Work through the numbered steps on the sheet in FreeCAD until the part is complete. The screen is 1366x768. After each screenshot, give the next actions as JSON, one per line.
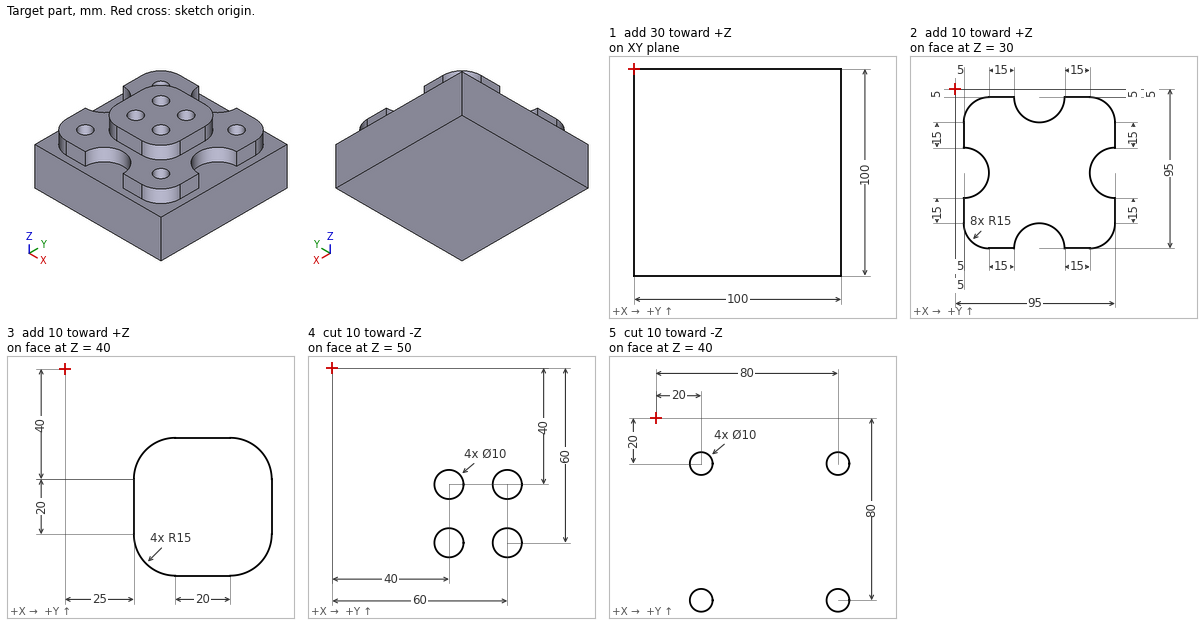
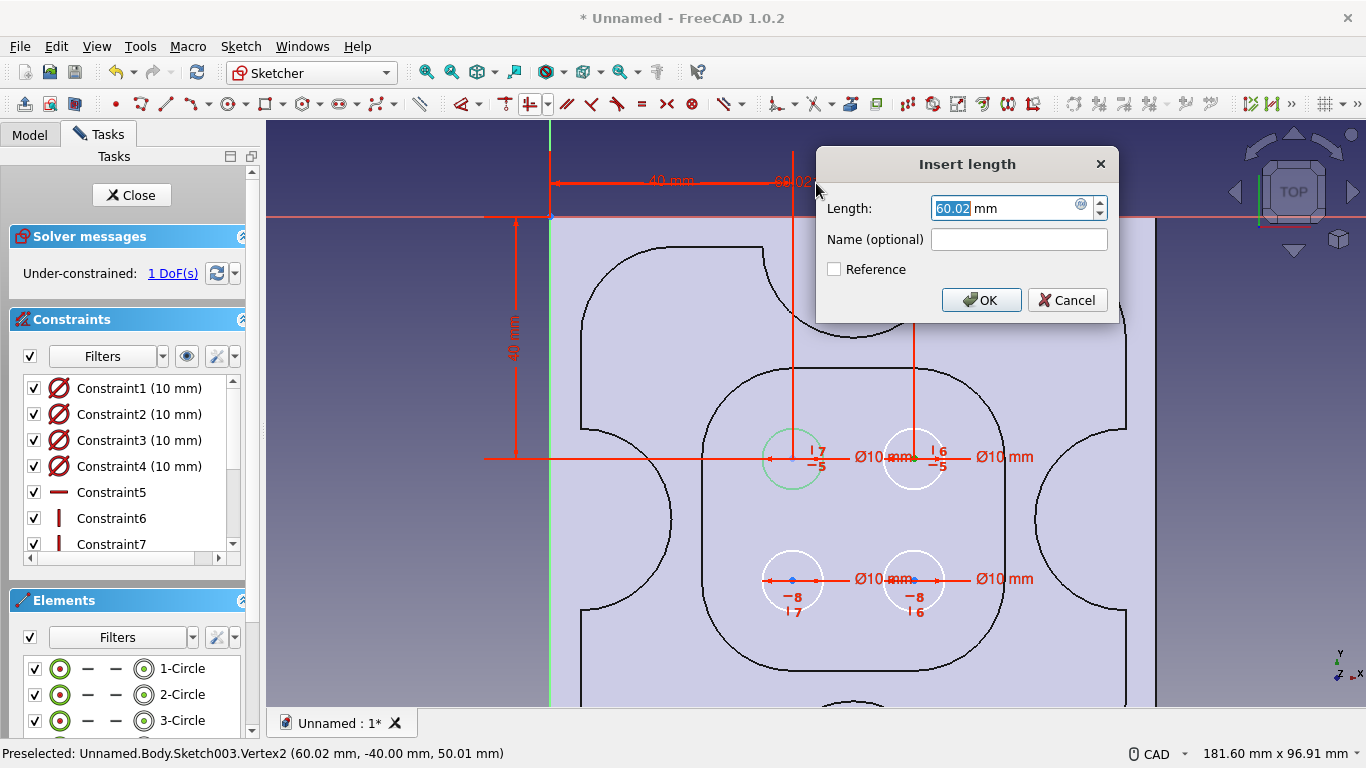
{"action": "type", "text": "60"}
{"action": "key", "text": "Return"}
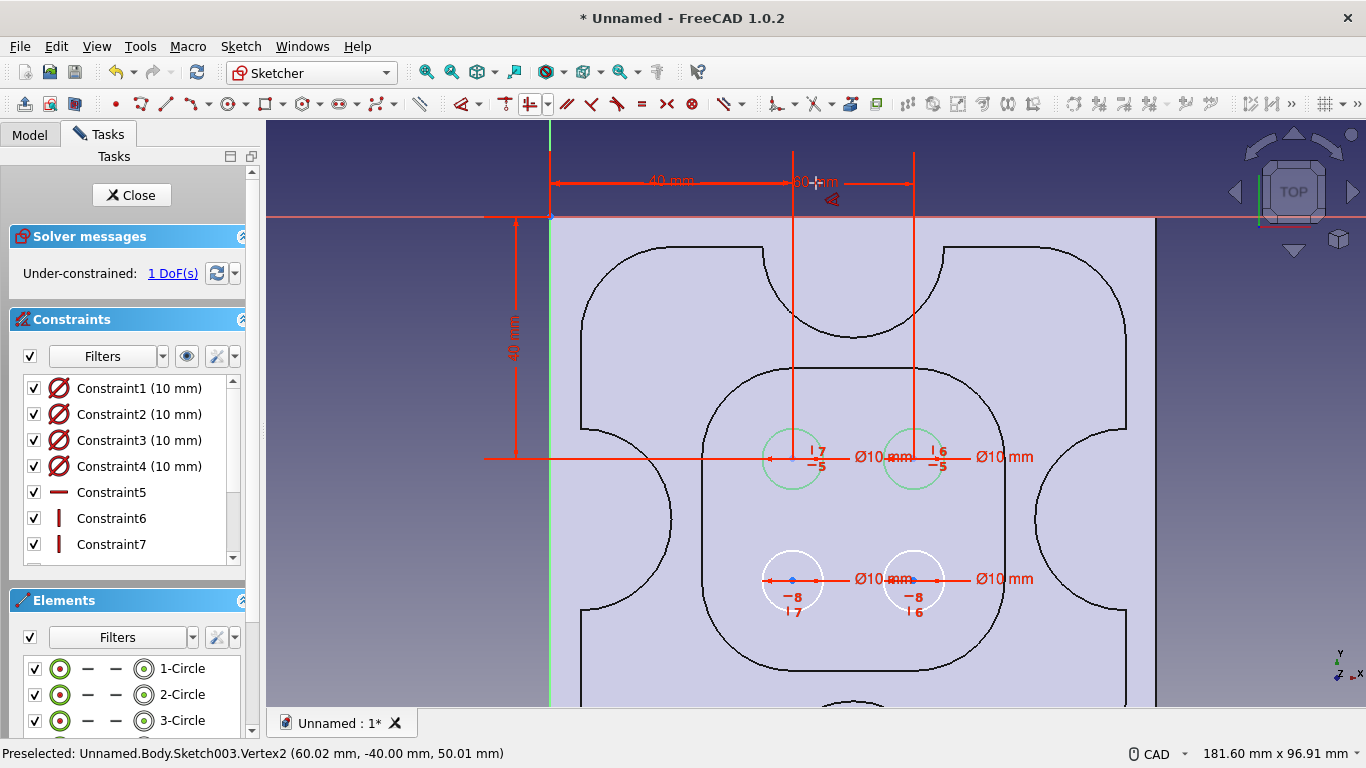
{"action": "left_click", "coordinate": [914, 581]}
{"action": "left_click", "coordinate": [516, 399]}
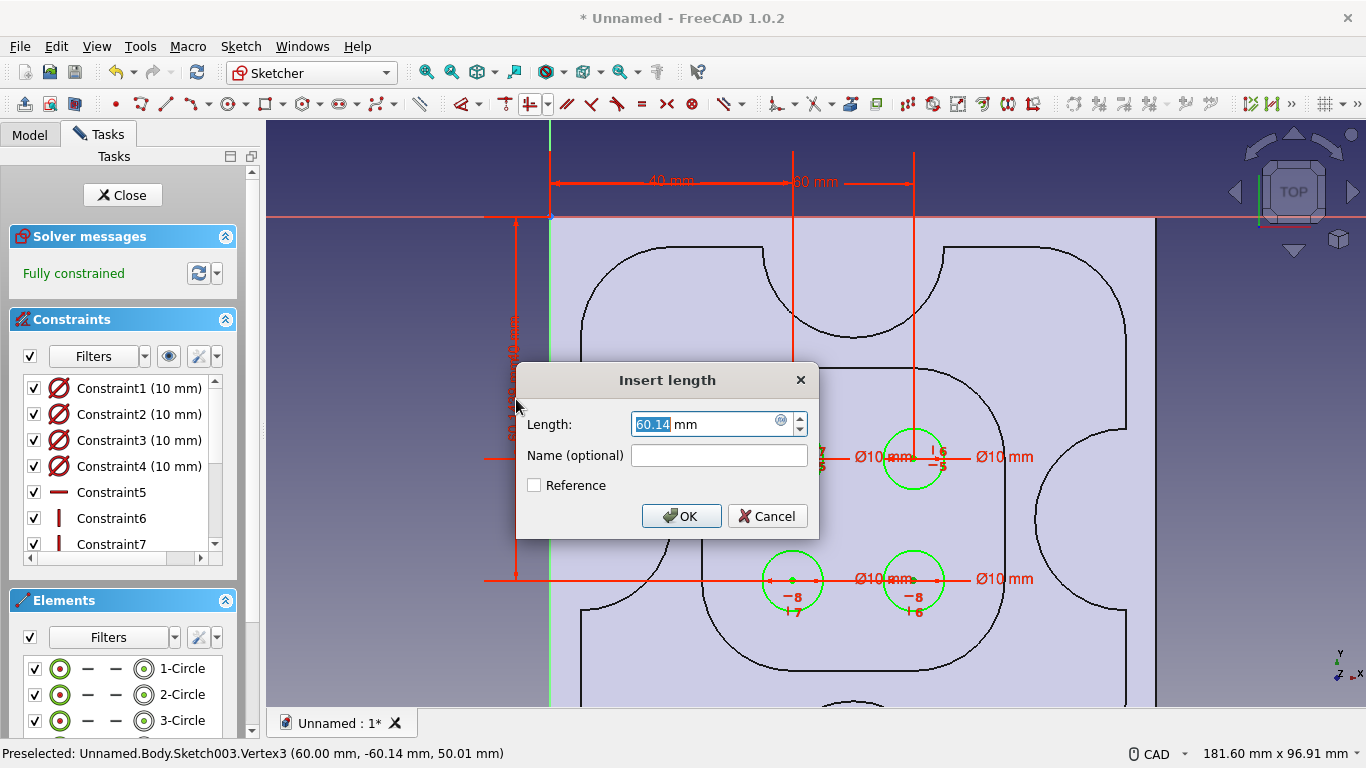
{"action": "type", "text": "60"}
{"action": "key", "text": "Return"}
{"action": "key", "text": "Escape"}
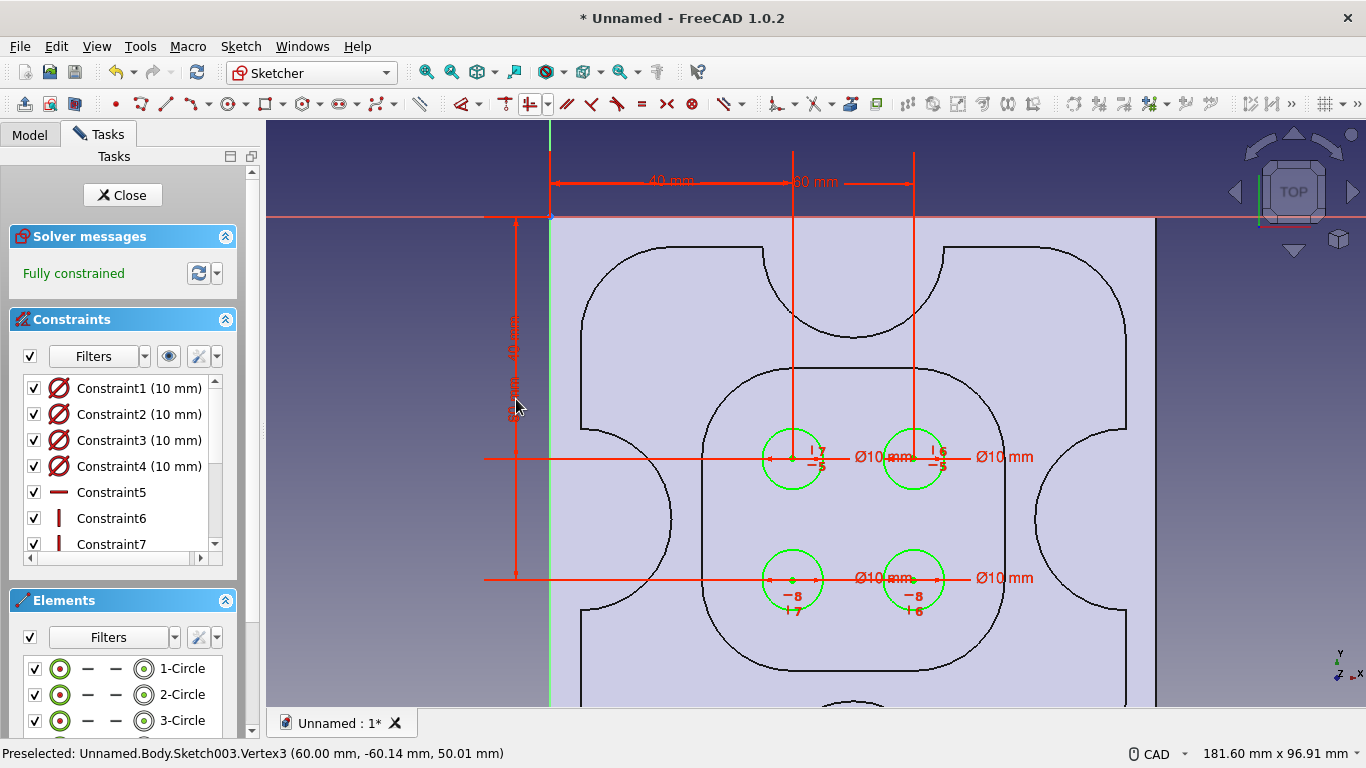
{"action": "left_click", "coordinate": [123, 195]}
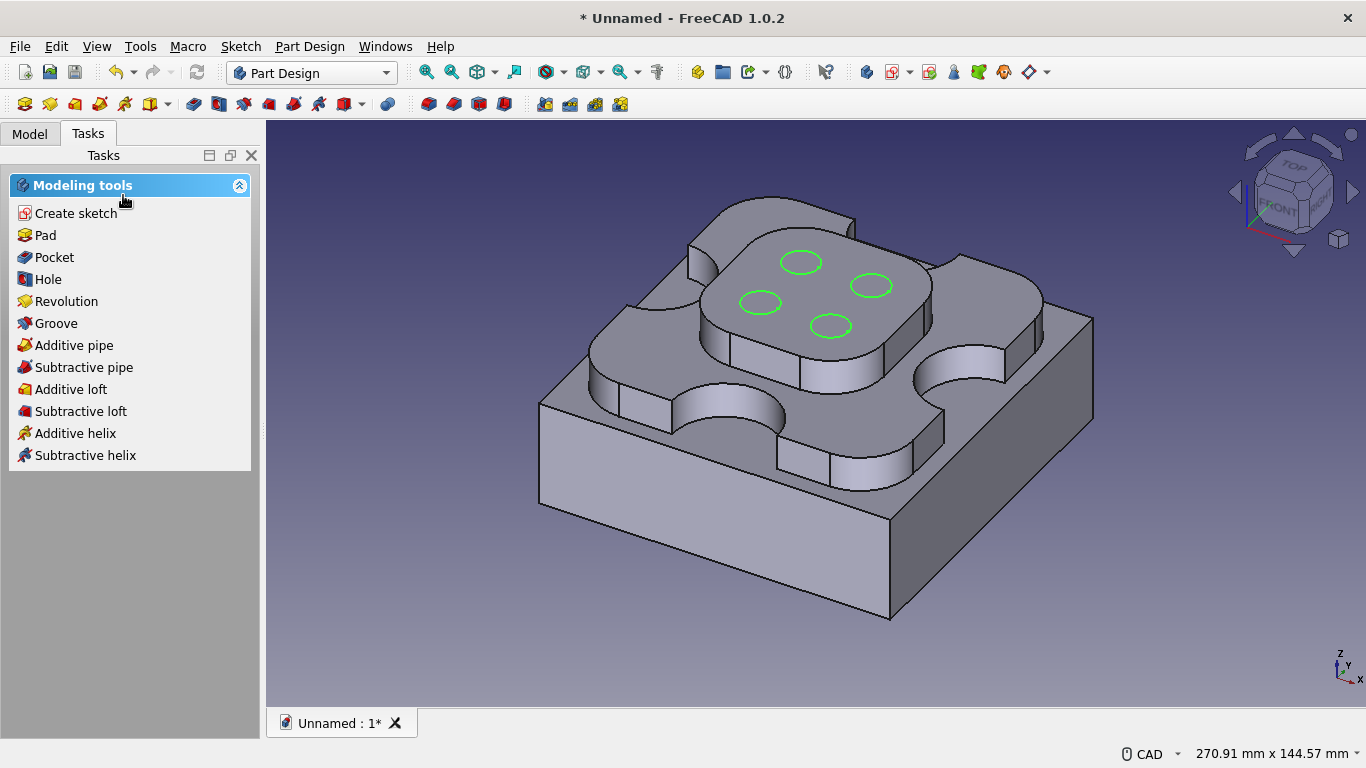
{"action": "left_click", "coordinate": [194, 104]}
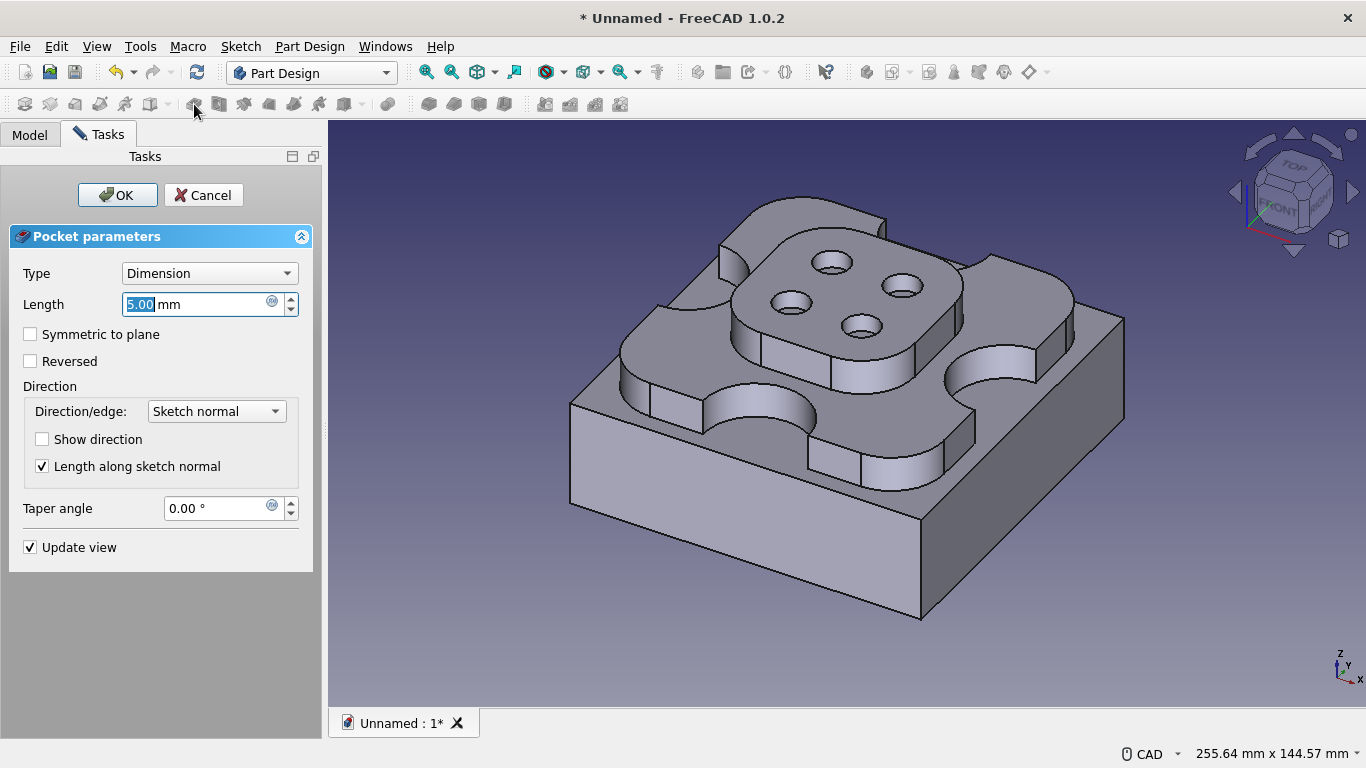
{"action": "type", "text": "10"}
{"action": "key", "text": "Tab"}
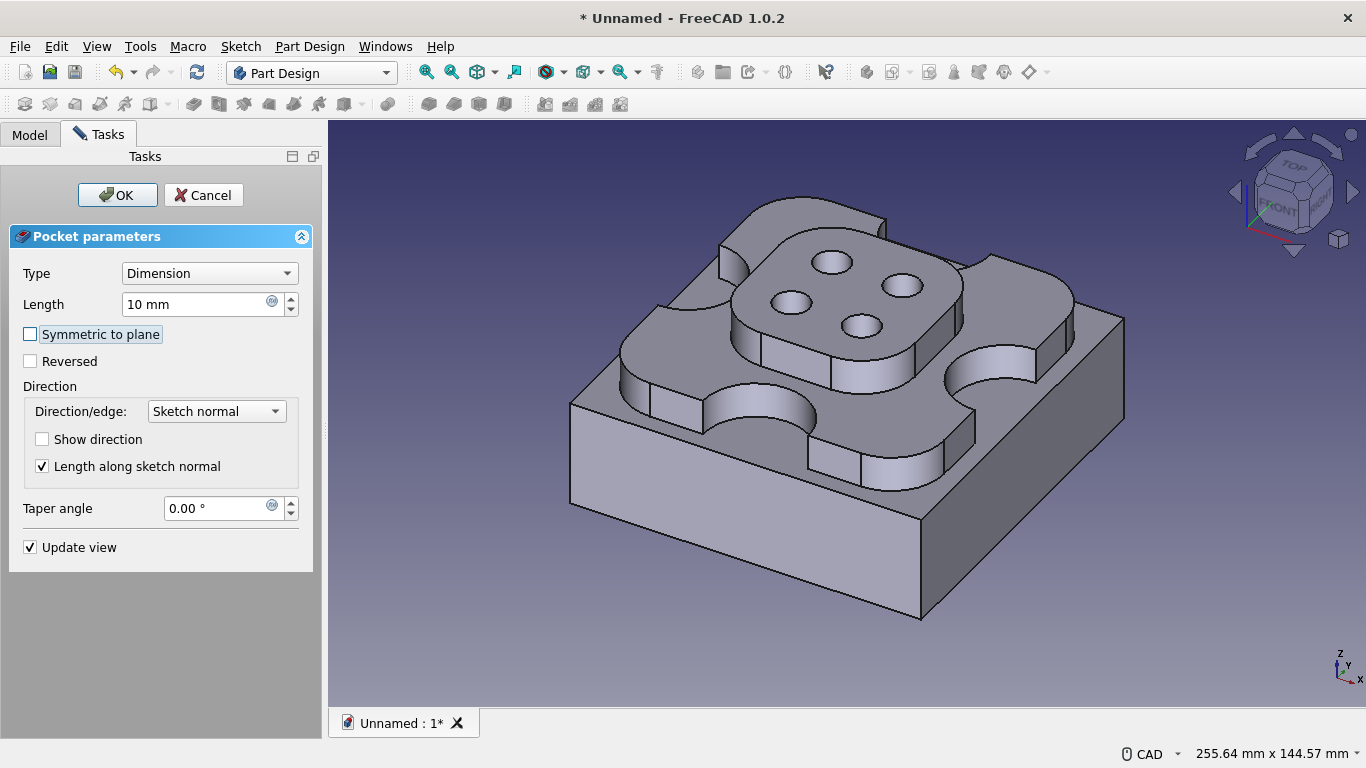
{"action": "left_click", "coordinate": [118, 195]}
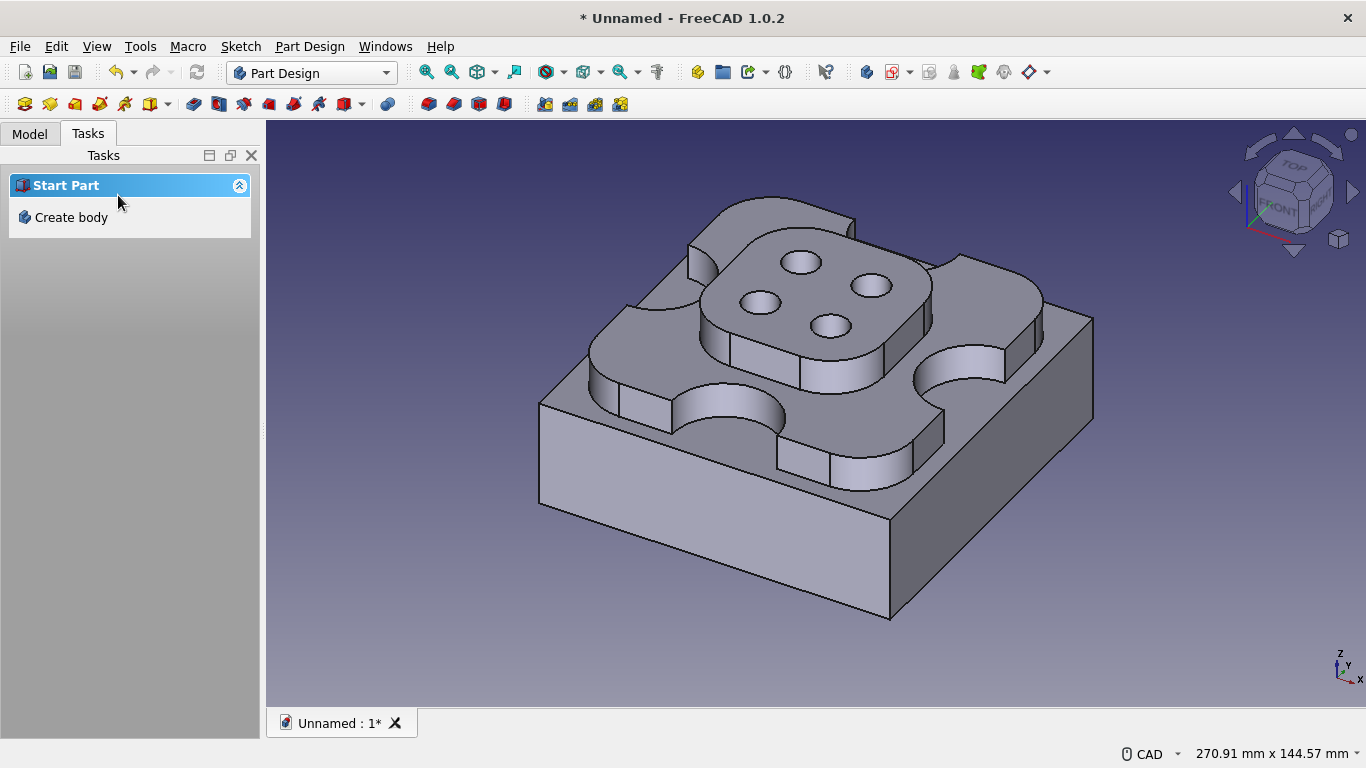
{"action": "left_click", "coordinate": [959, 305]}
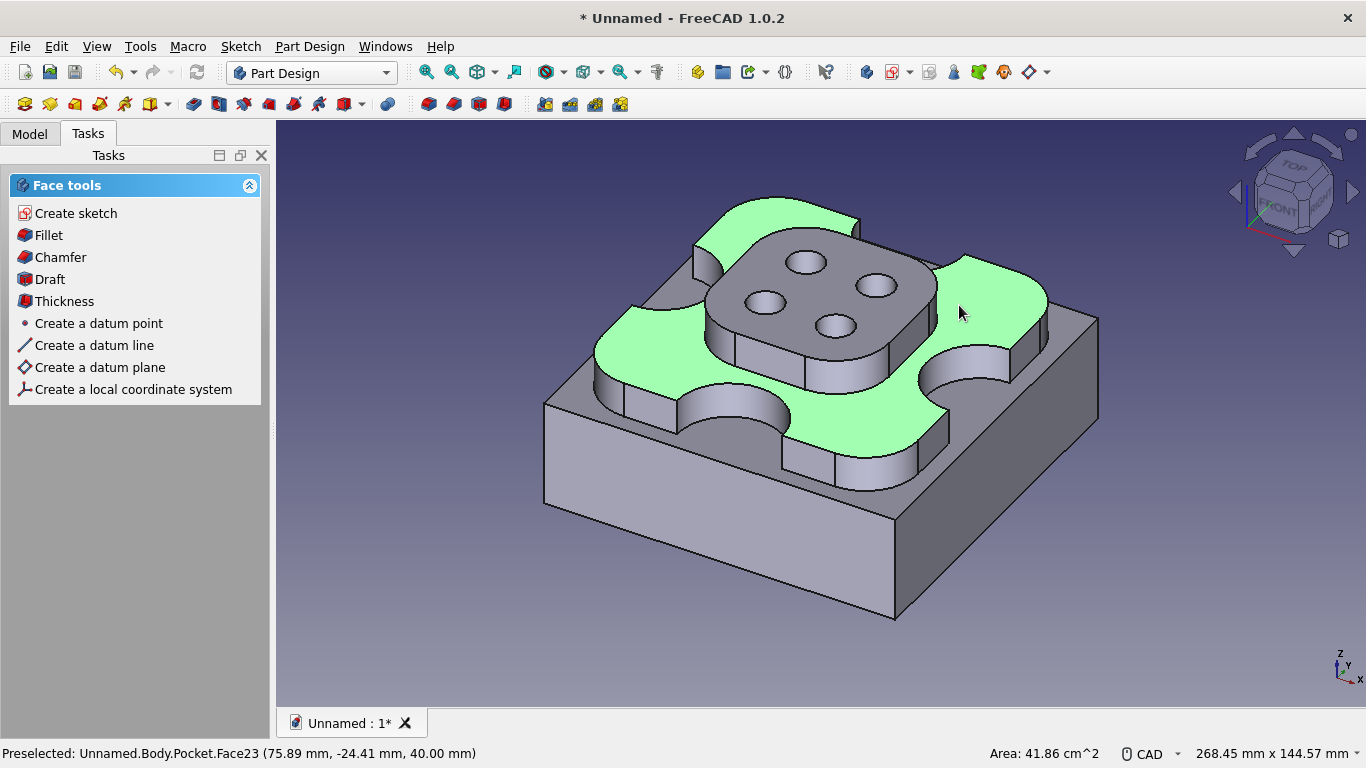
{"action": "left_click", "coordinate": [892, 72]}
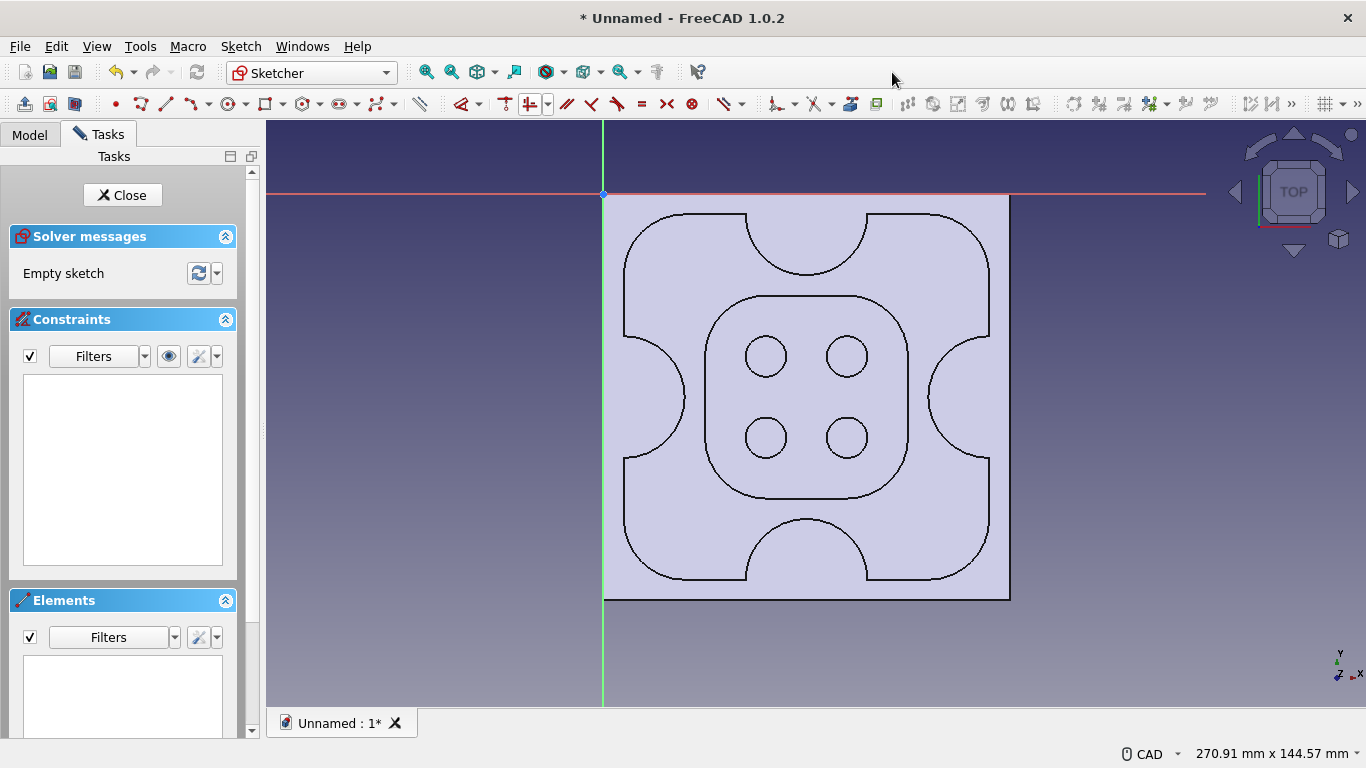
{"action": "key", "text": "g c"}